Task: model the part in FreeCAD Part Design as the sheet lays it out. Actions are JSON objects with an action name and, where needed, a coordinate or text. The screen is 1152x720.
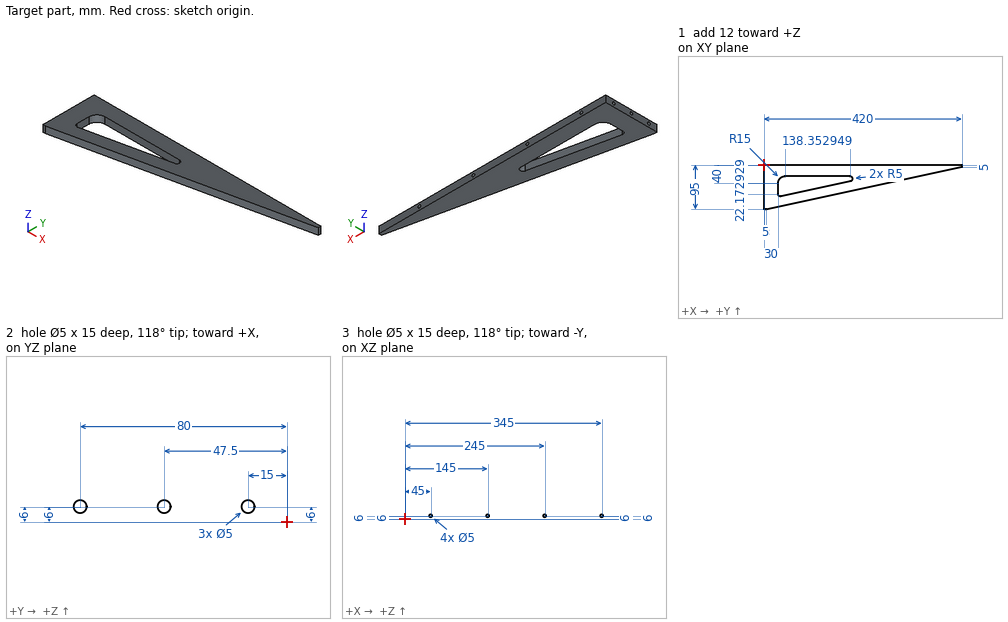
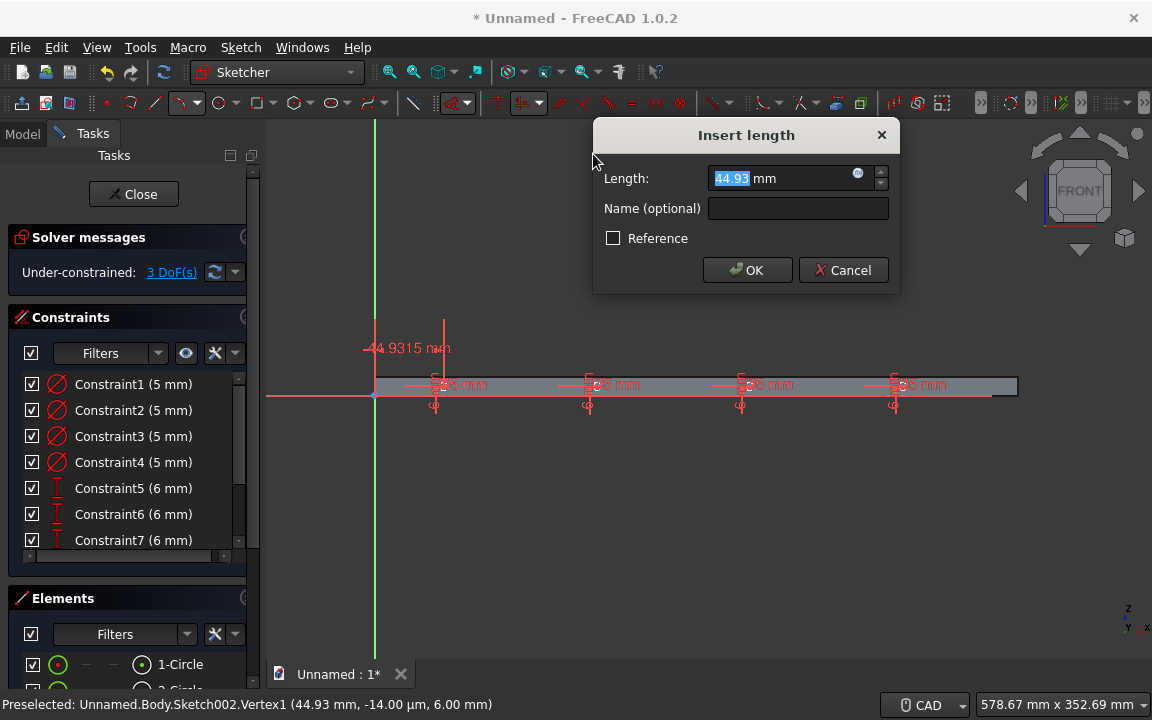
{"action": "type", "text": "45"}
{"action": "key", "text": "Return"}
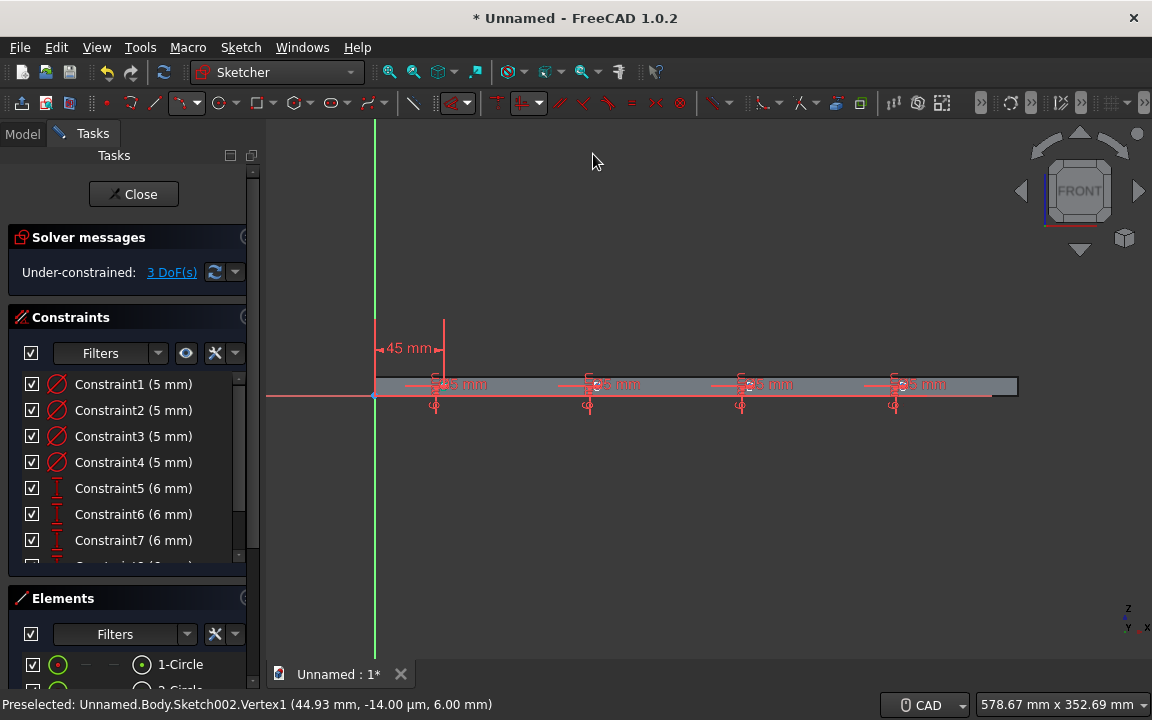
{"action": "left_click", "coordinate": [597, 386]}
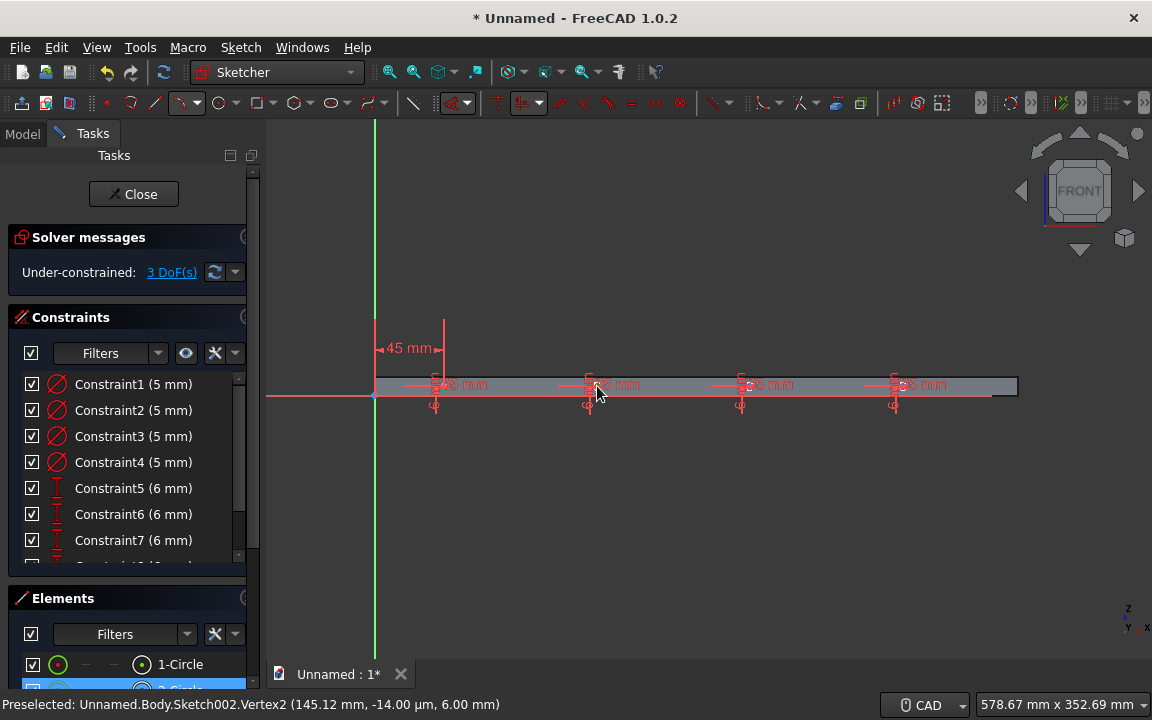
{"action": "left_click", "coordinate": [470, 104]}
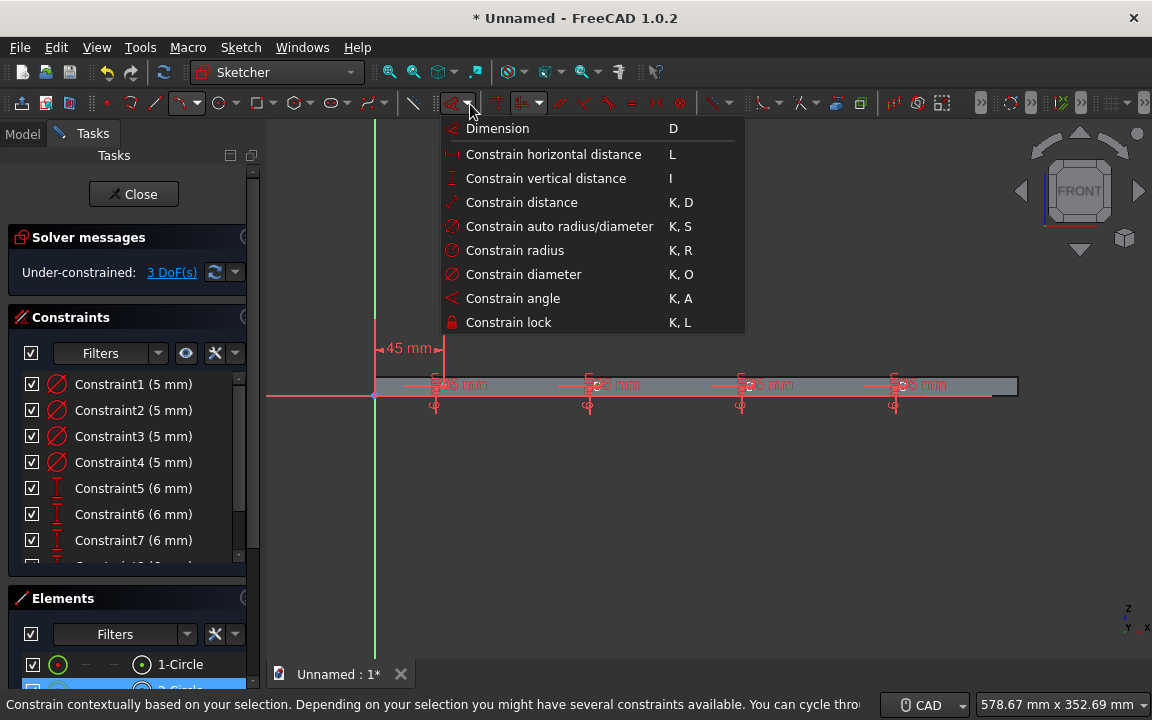
{"action": "left_click", "coordinate": [593, 154]}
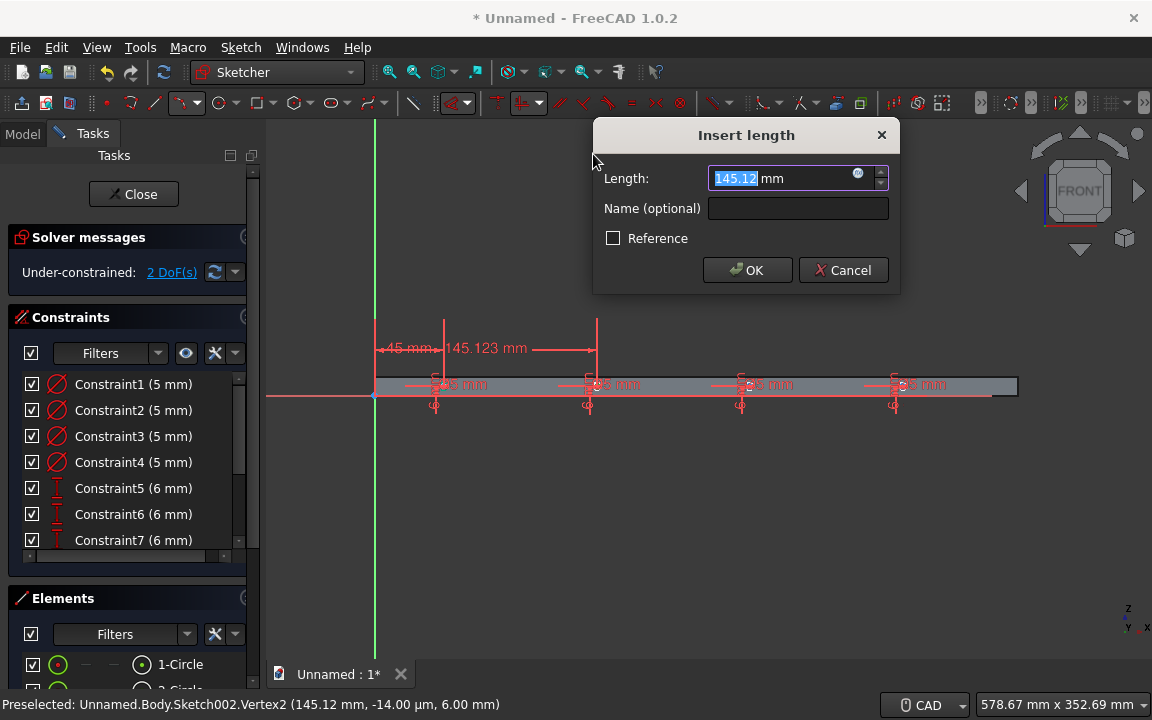
{"action": "type", "text": "145"}
{"action": "key", "text": "Return"}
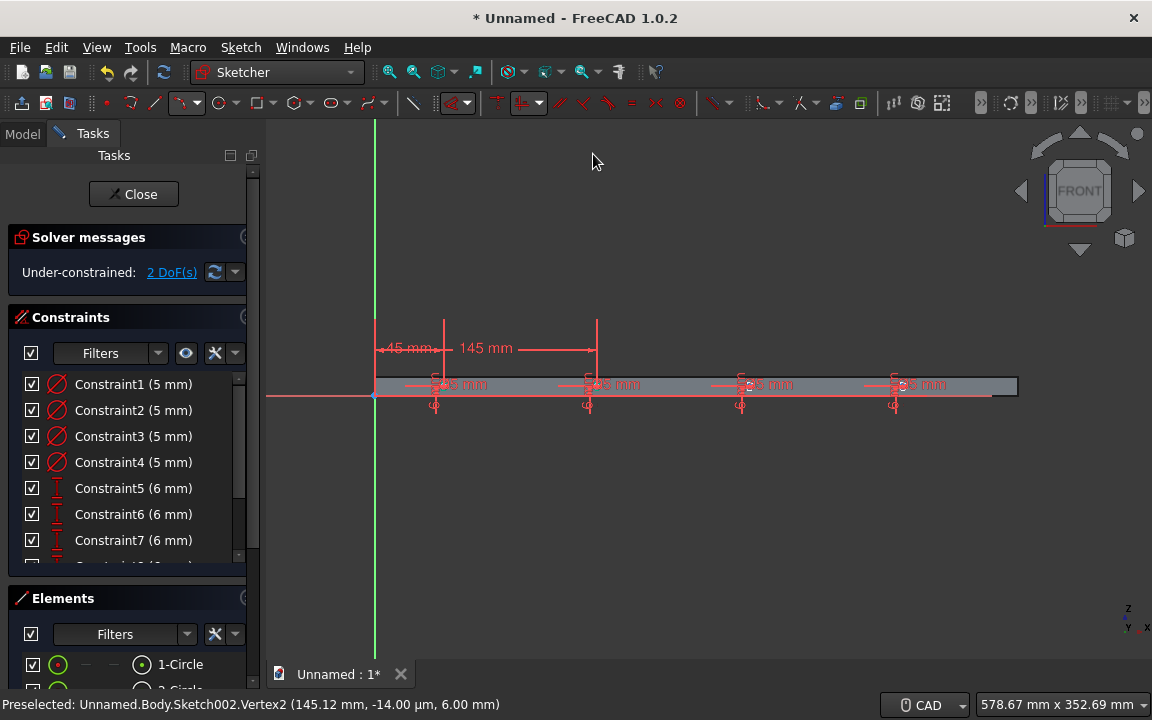
{"action": "left_click", "coordinate": [750, 386]}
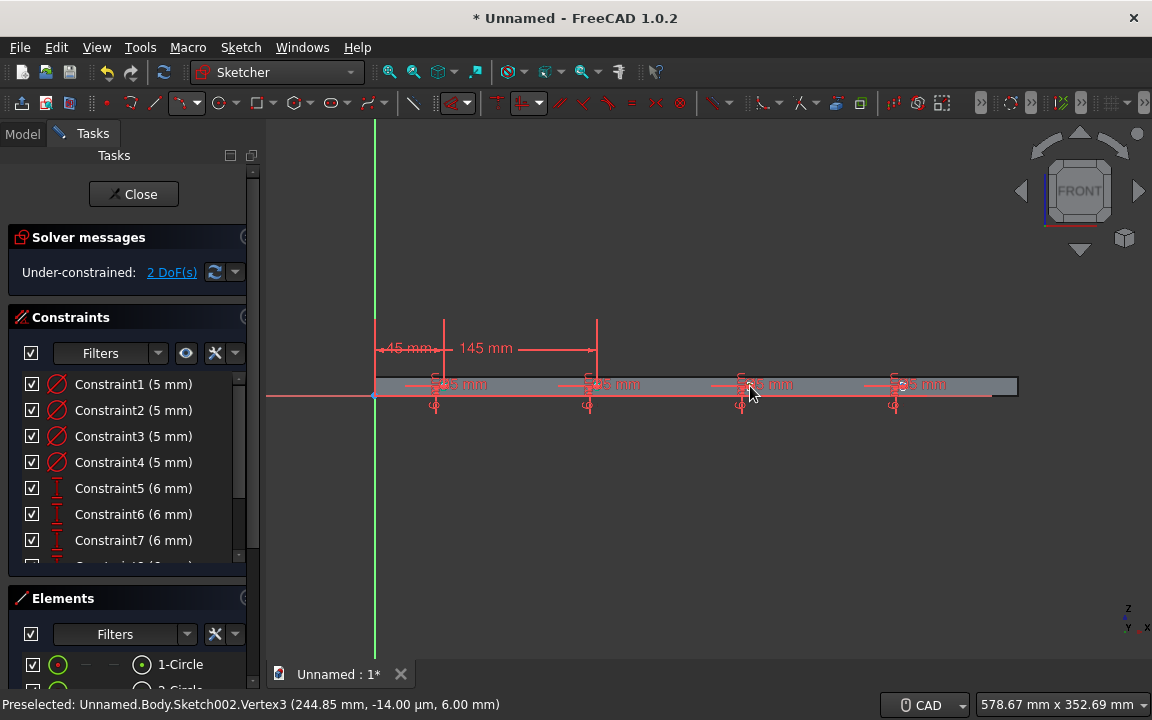
{"action": "left_click", "coordinate": [470, 104]}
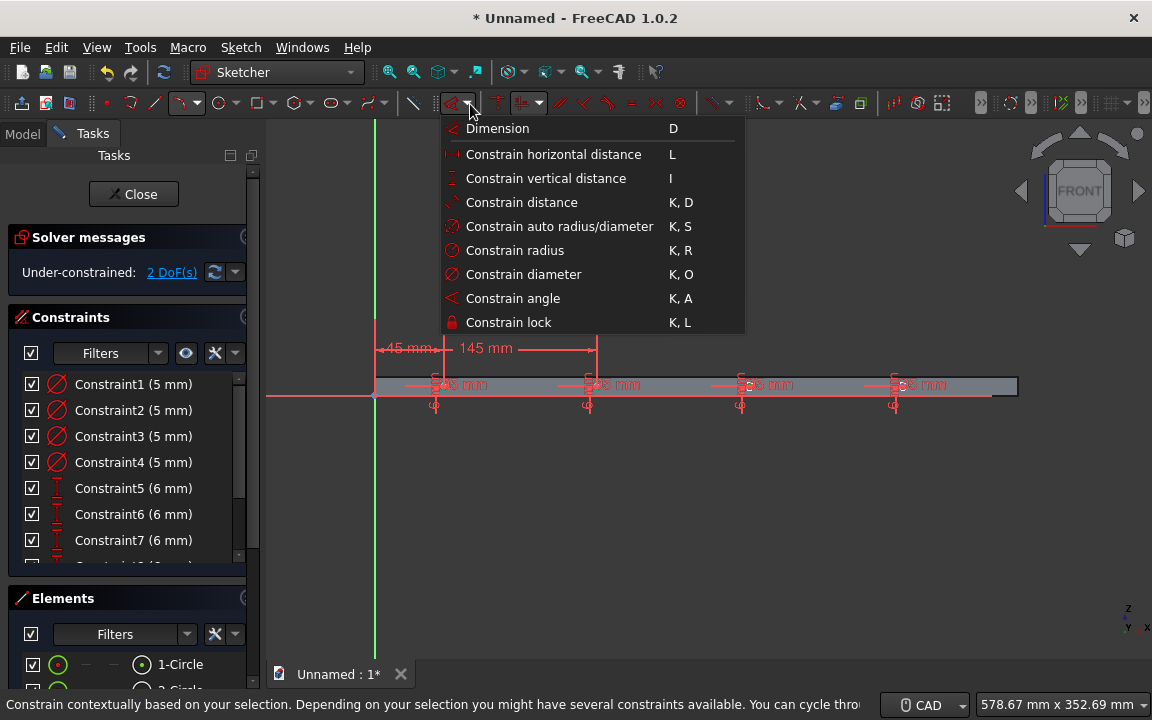
{"action": "left_click", "coordinate": [593, 154]}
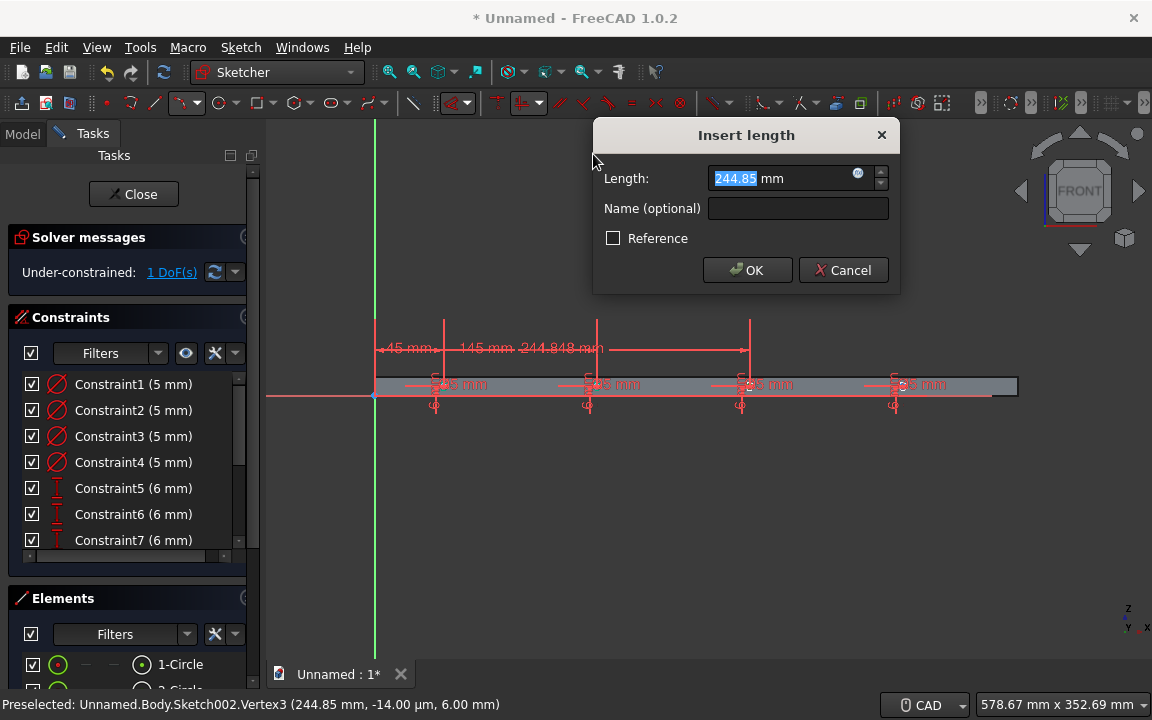
{"action": "type", "text": "245"}
{"action": "key", "text": "Return"}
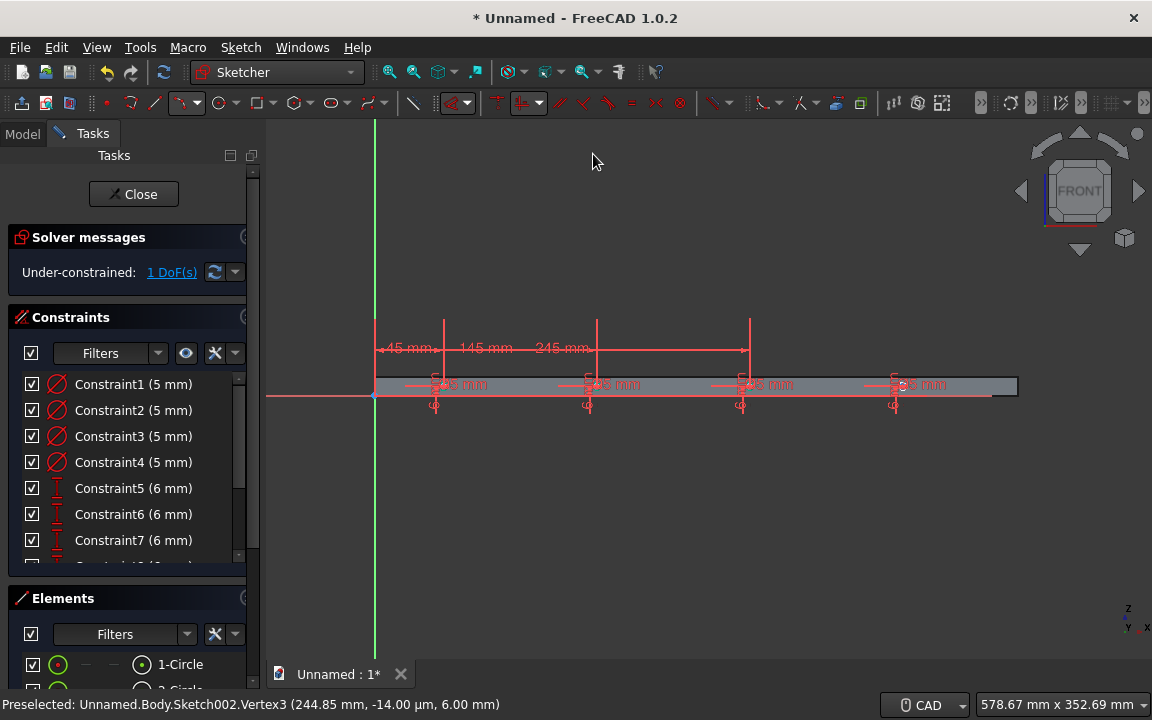
{"action": "left_click", "coordinate": [903, 386]}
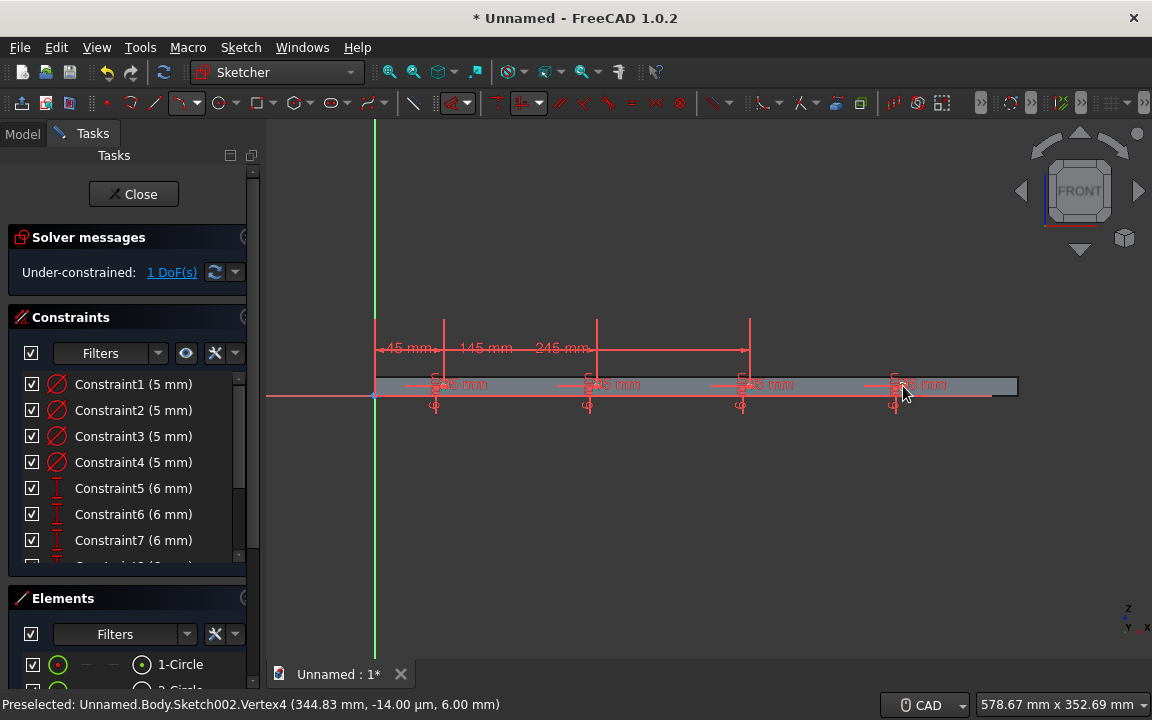
{"action": "left_click", "coordinate": [470, 104]}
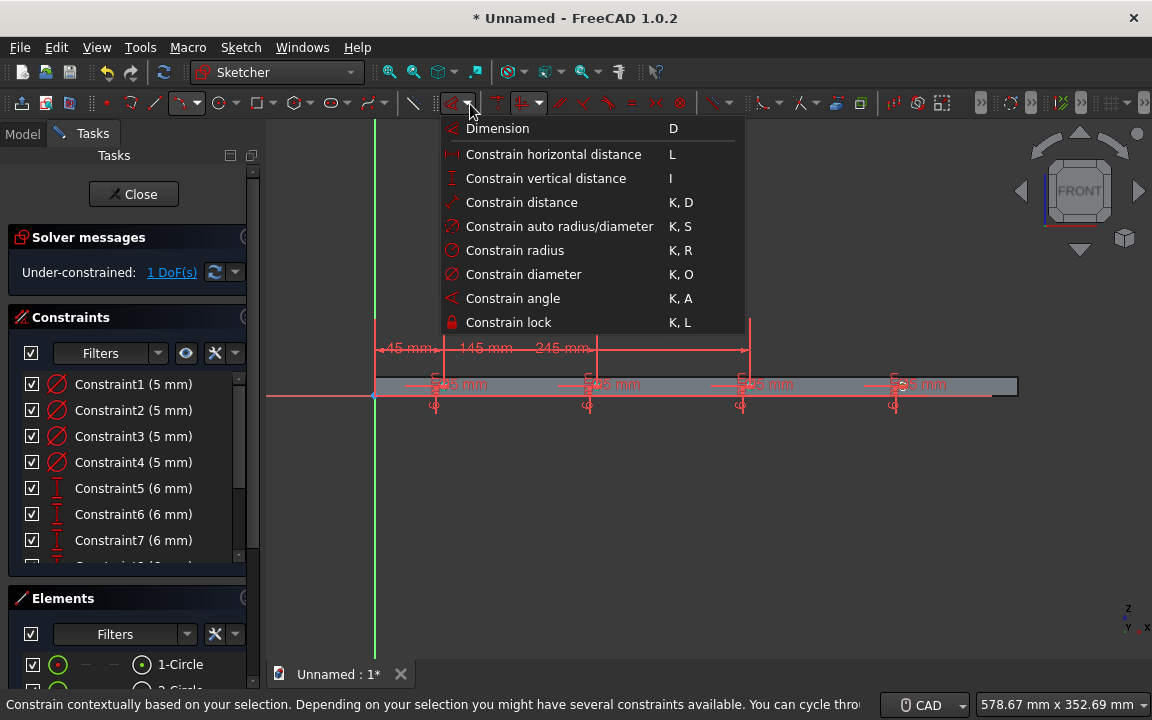
{"action": "left_click", "coordinate": [593, 154]}